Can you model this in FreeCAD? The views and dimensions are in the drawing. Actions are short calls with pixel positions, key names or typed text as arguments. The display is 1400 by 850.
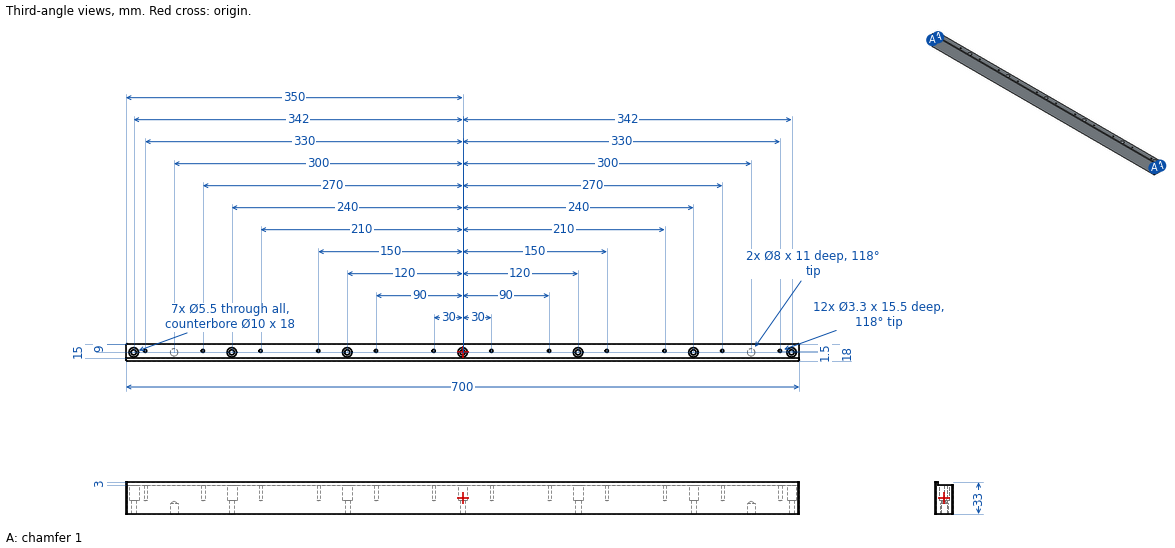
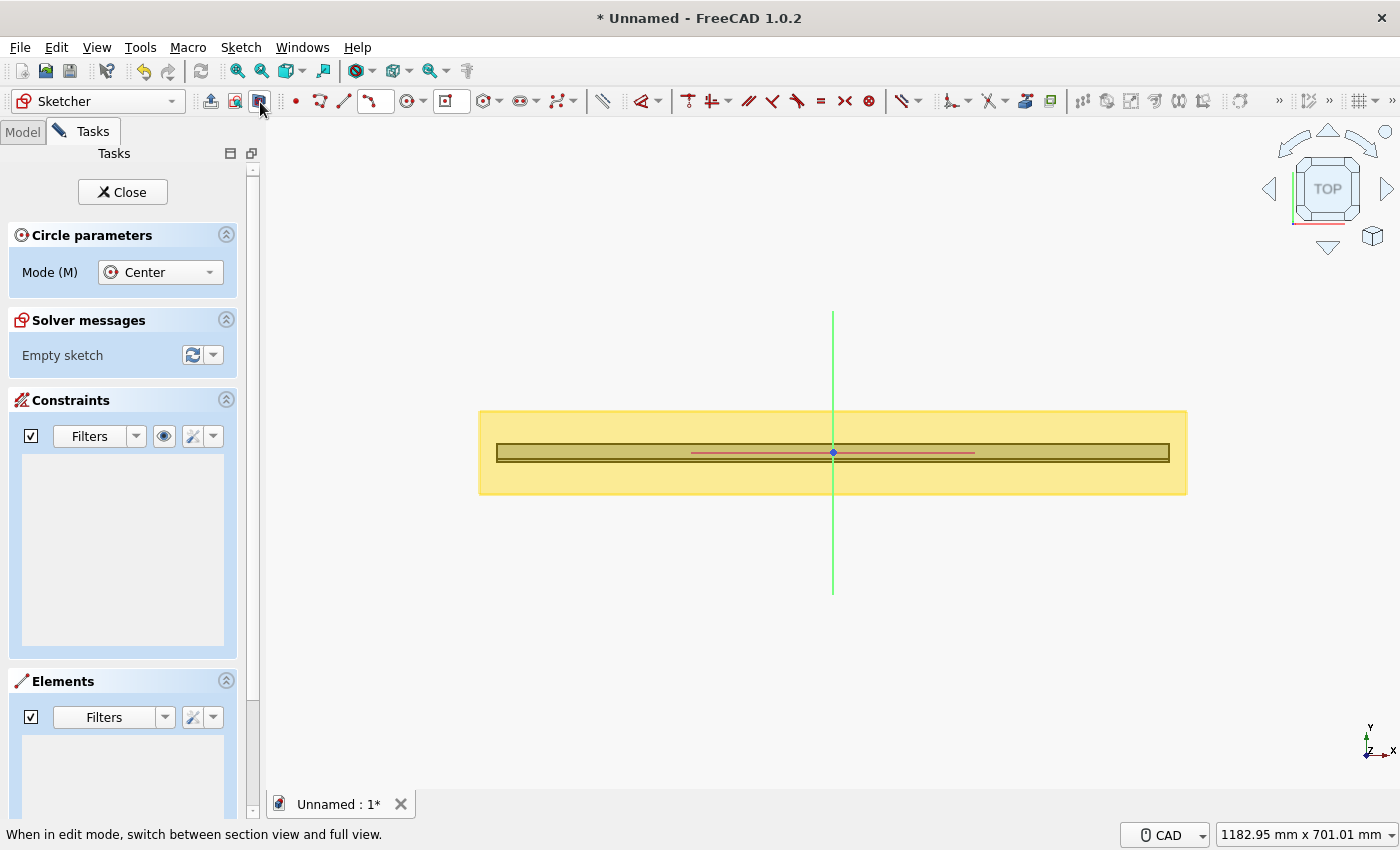
scroll(1149, 452, up, 14)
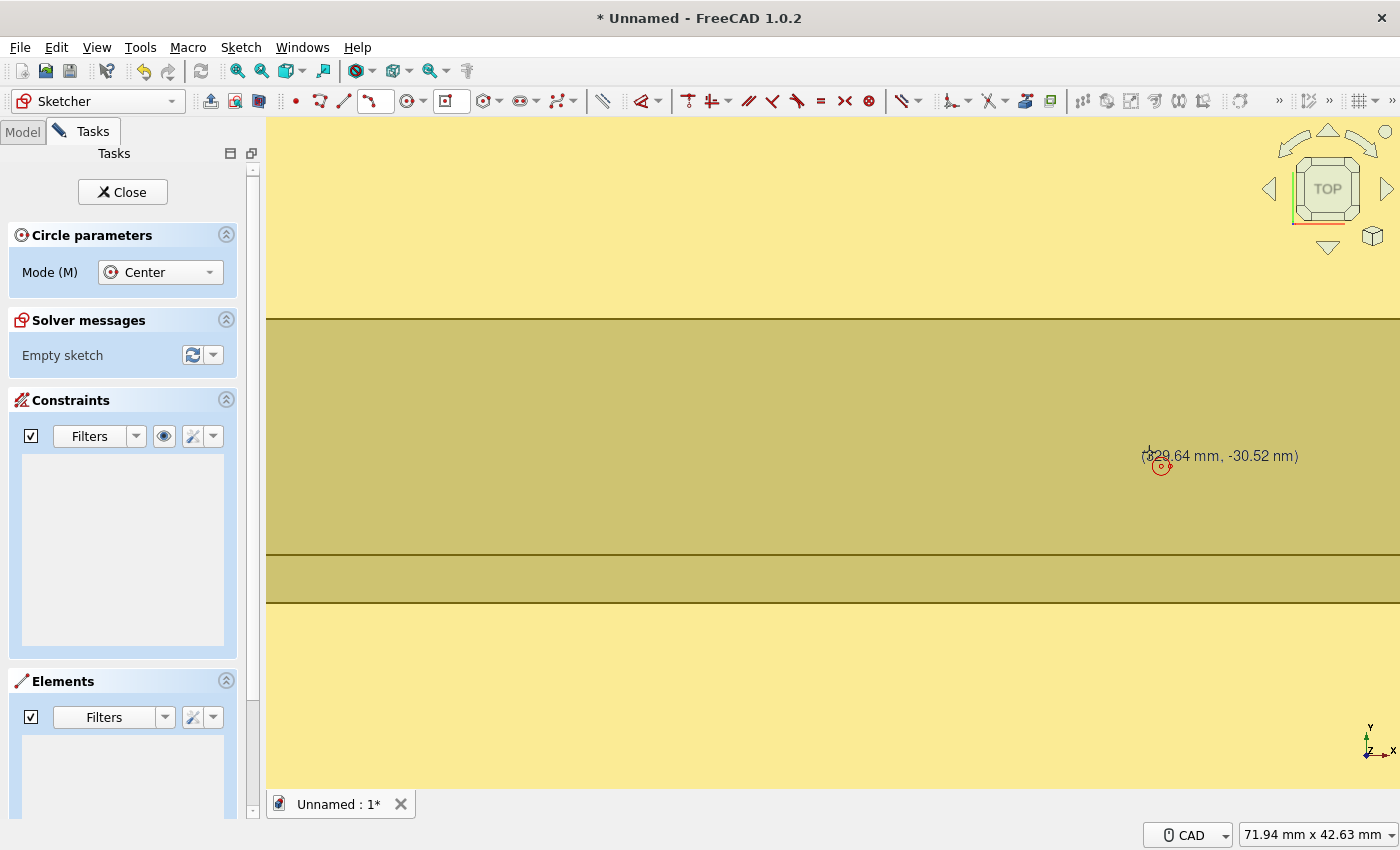
click(1143, 437)
click(1161, 419)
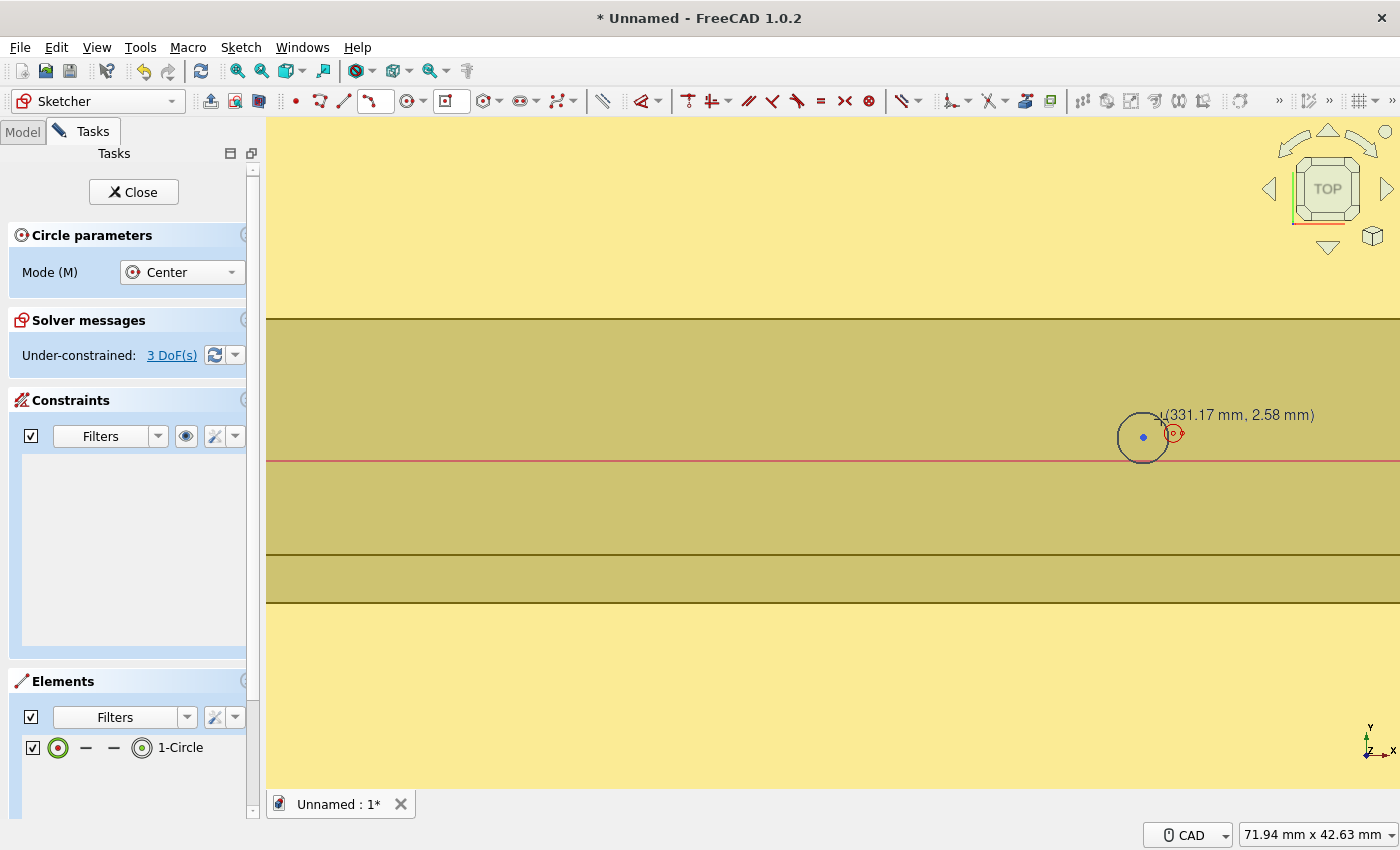
scroll(1077, 454, down, 14)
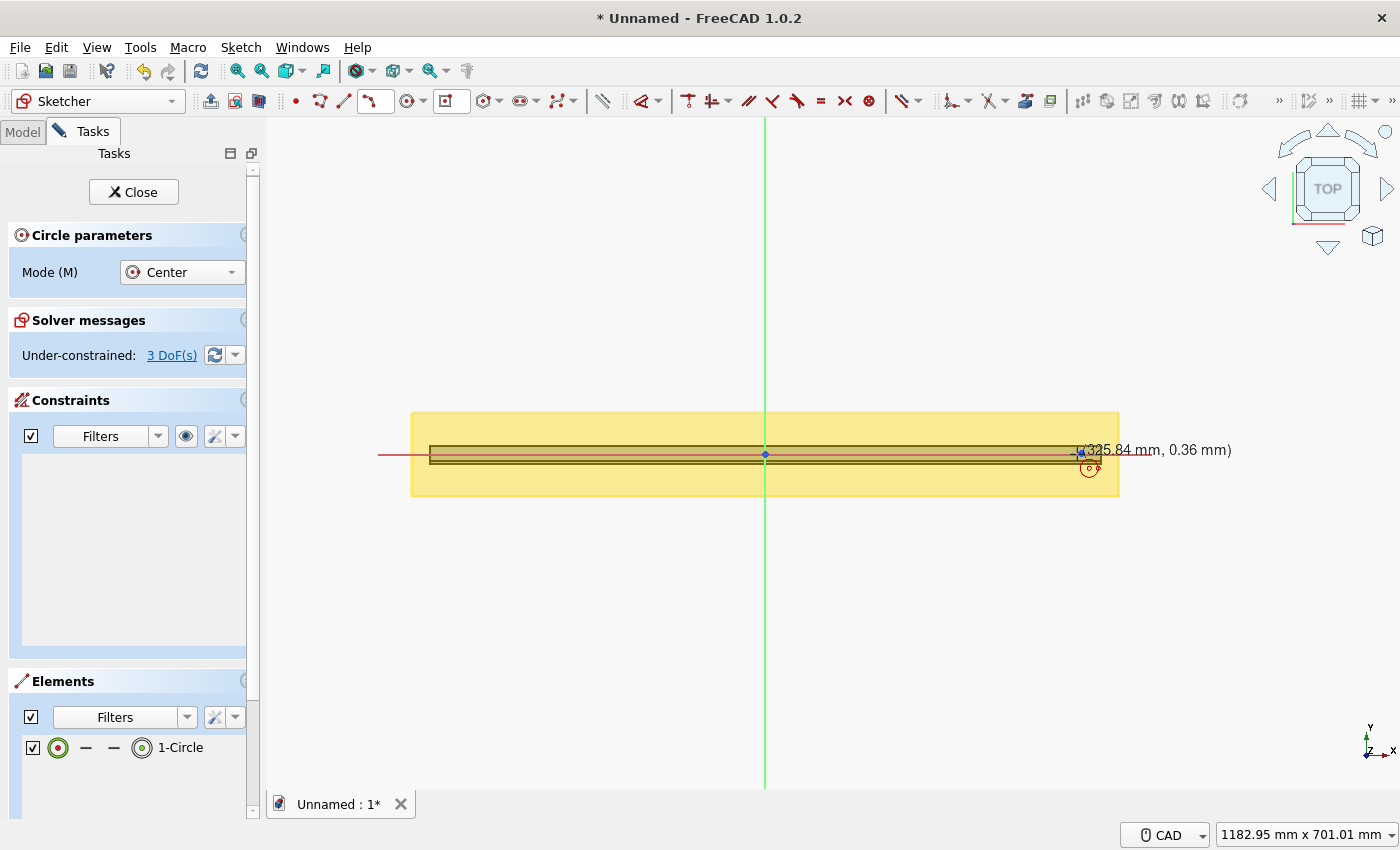
scroll(1024, 453, up, 14)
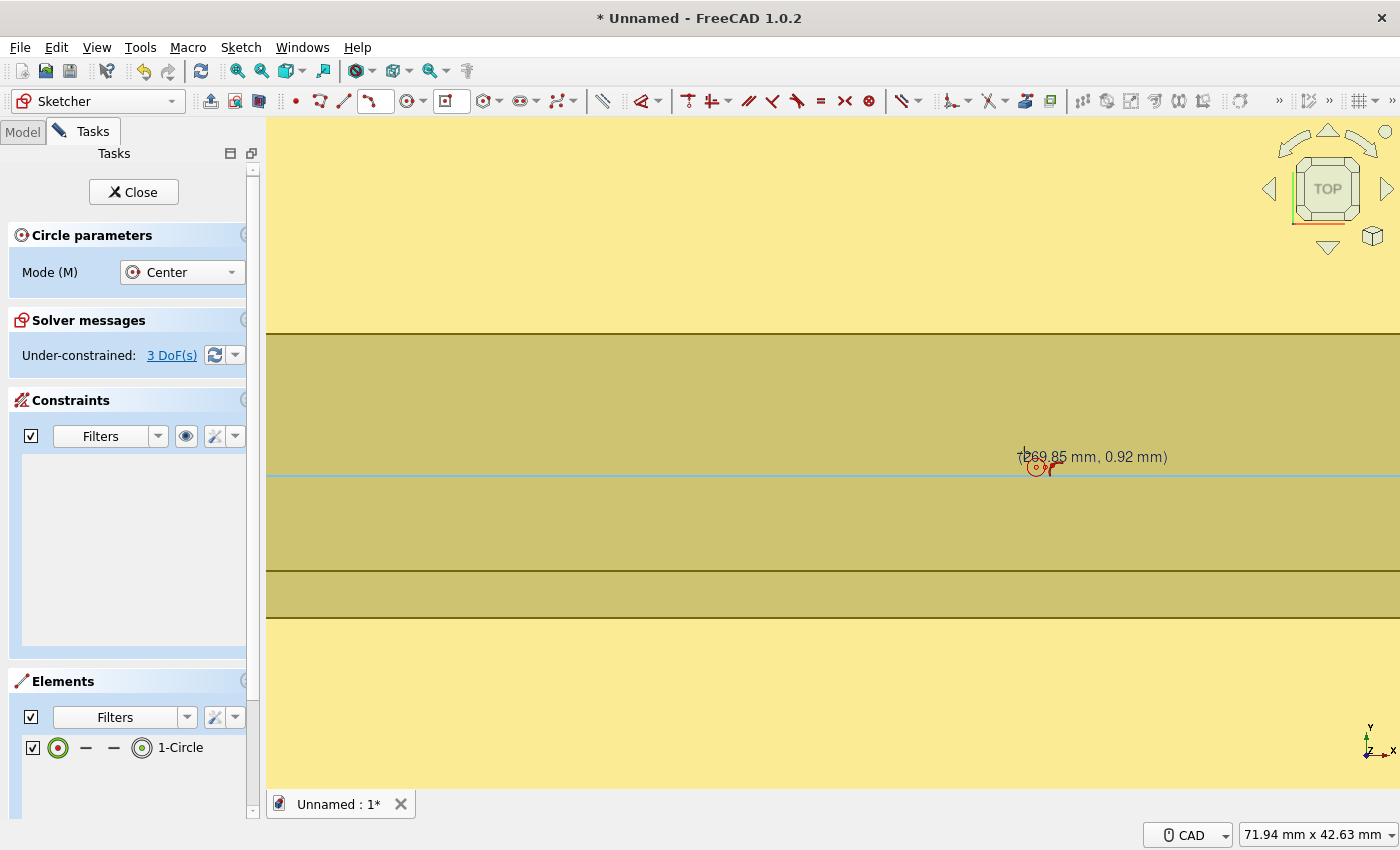
click(1016, 453)
click(1034, 434)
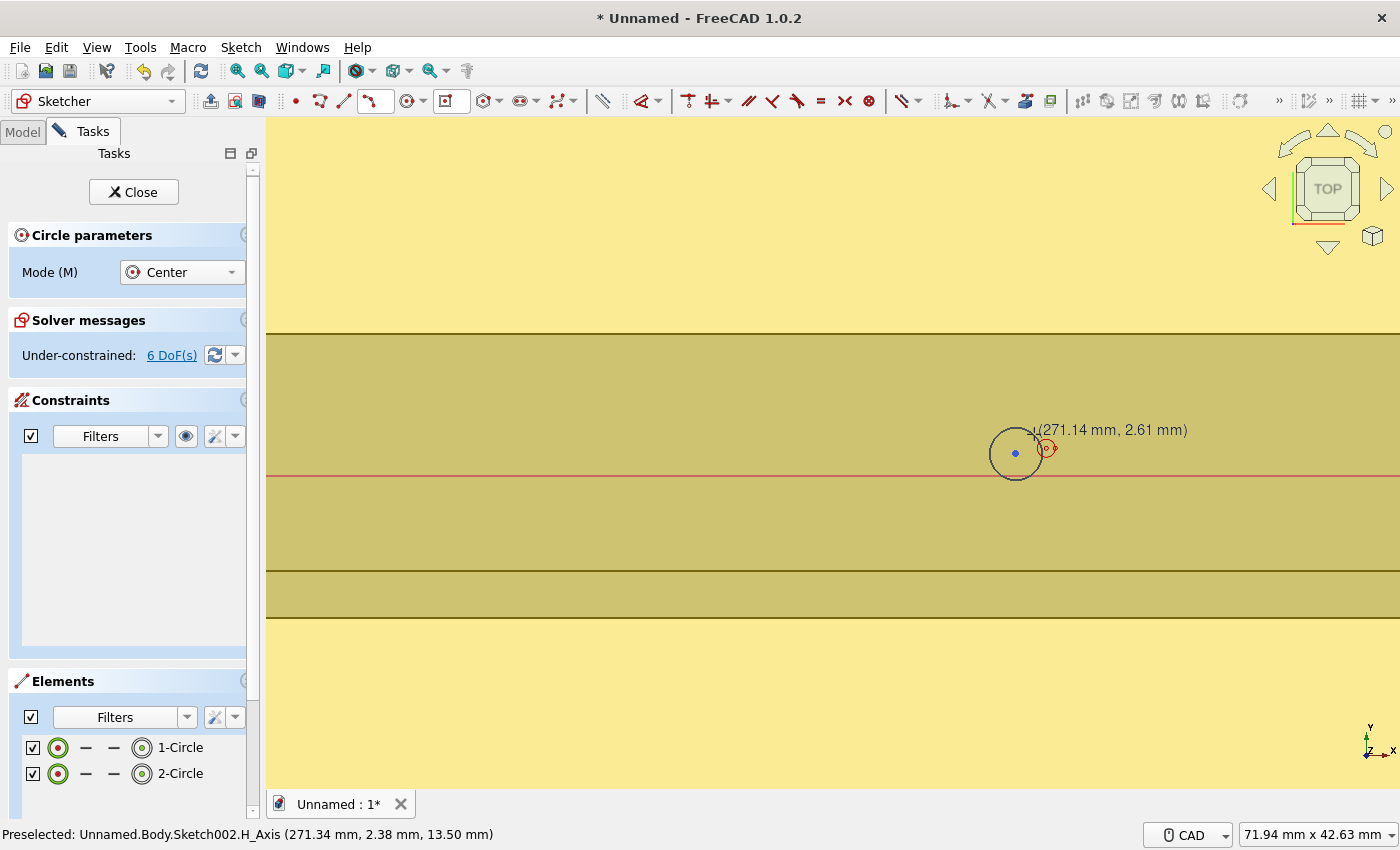
scroll(1024, 453, down, 14)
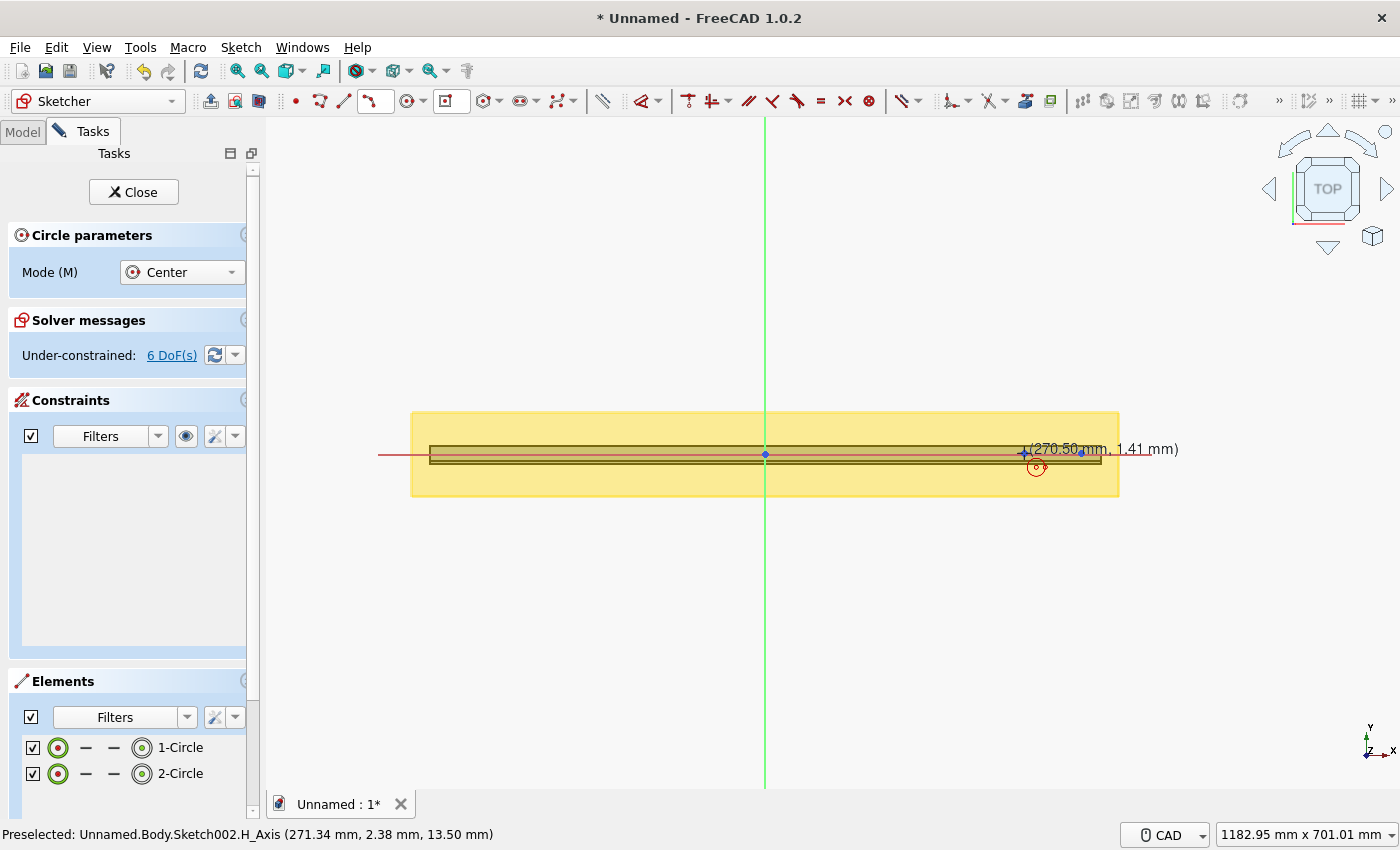
scroll(967, 453, up, 14)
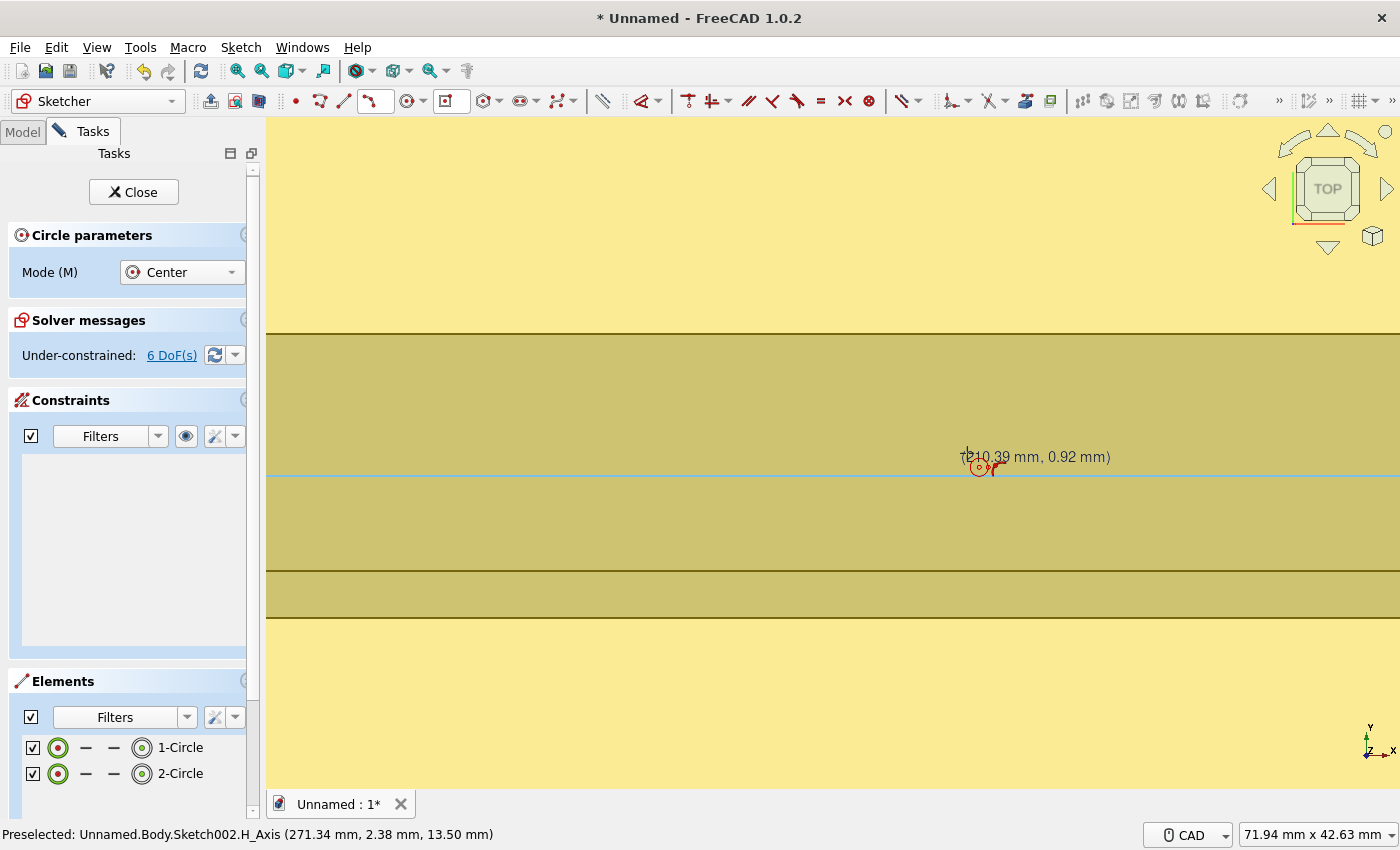
click(951, 453)
click(970, 434)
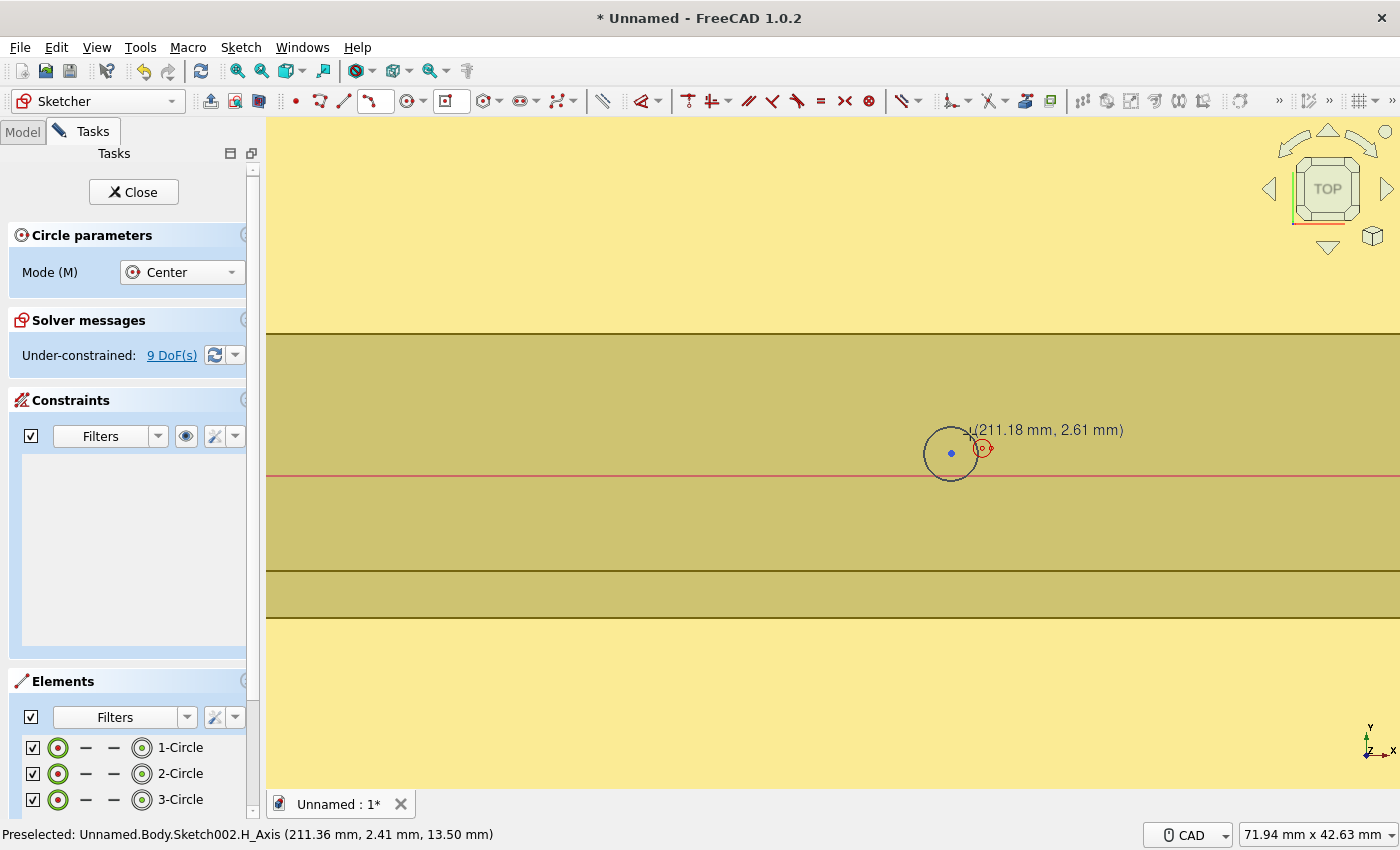
scroll(967, 453, down, 14)